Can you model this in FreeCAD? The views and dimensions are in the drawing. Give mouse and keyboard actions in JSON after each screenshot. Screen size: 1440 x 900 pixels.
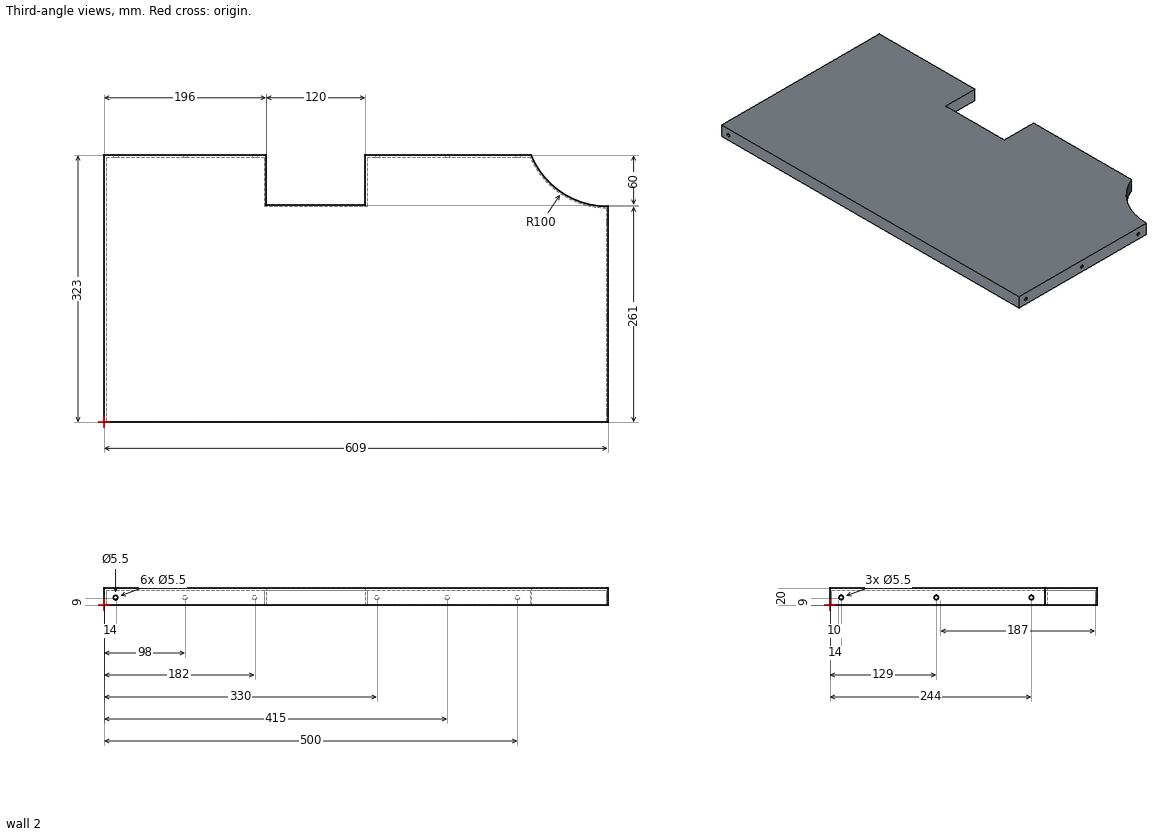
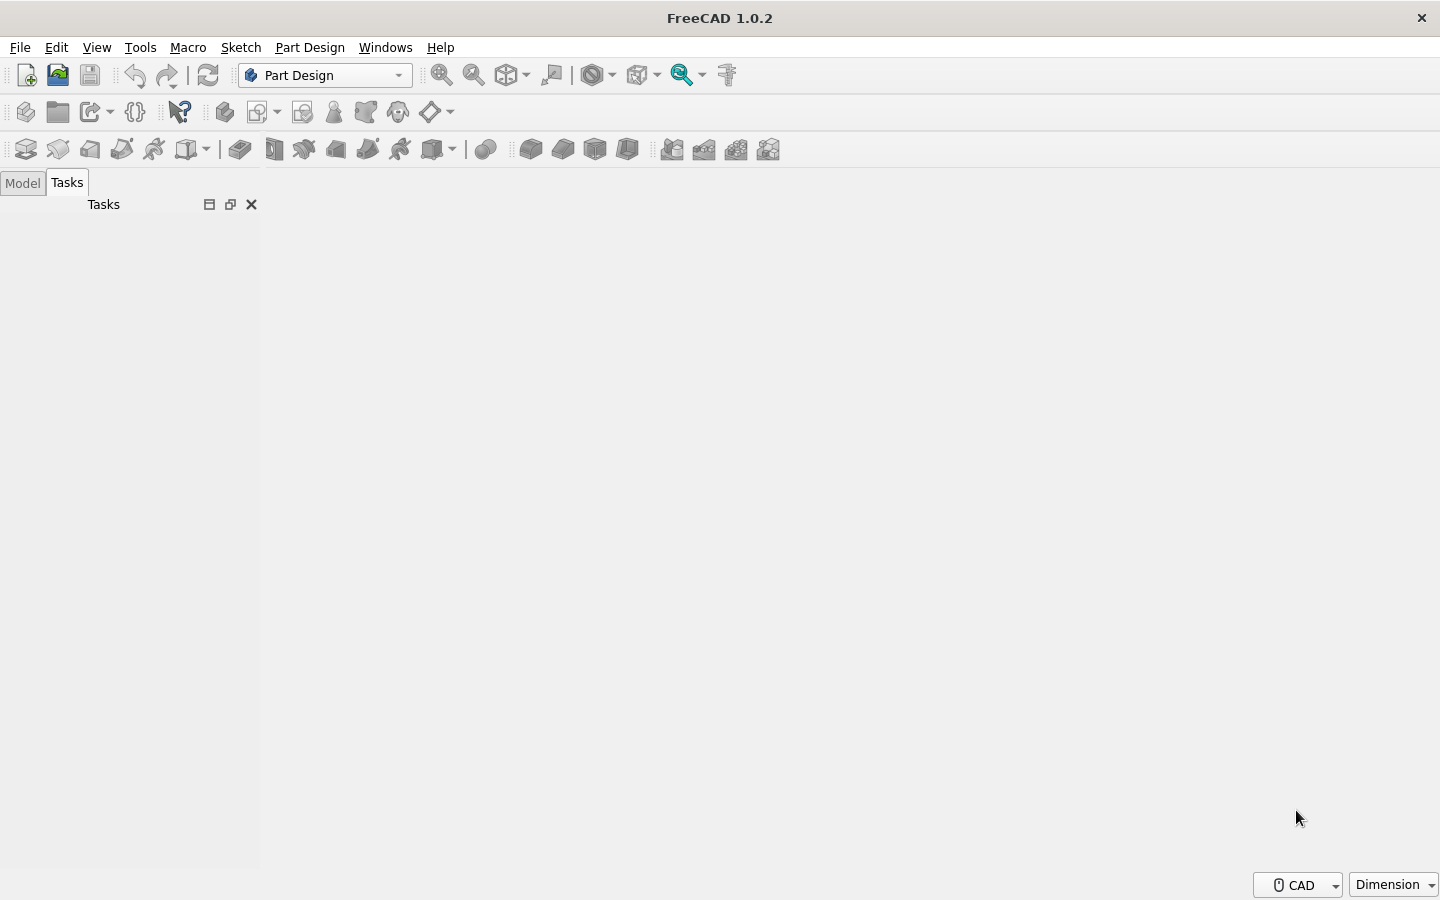
{"action": "key", "text": "ctrl+n"}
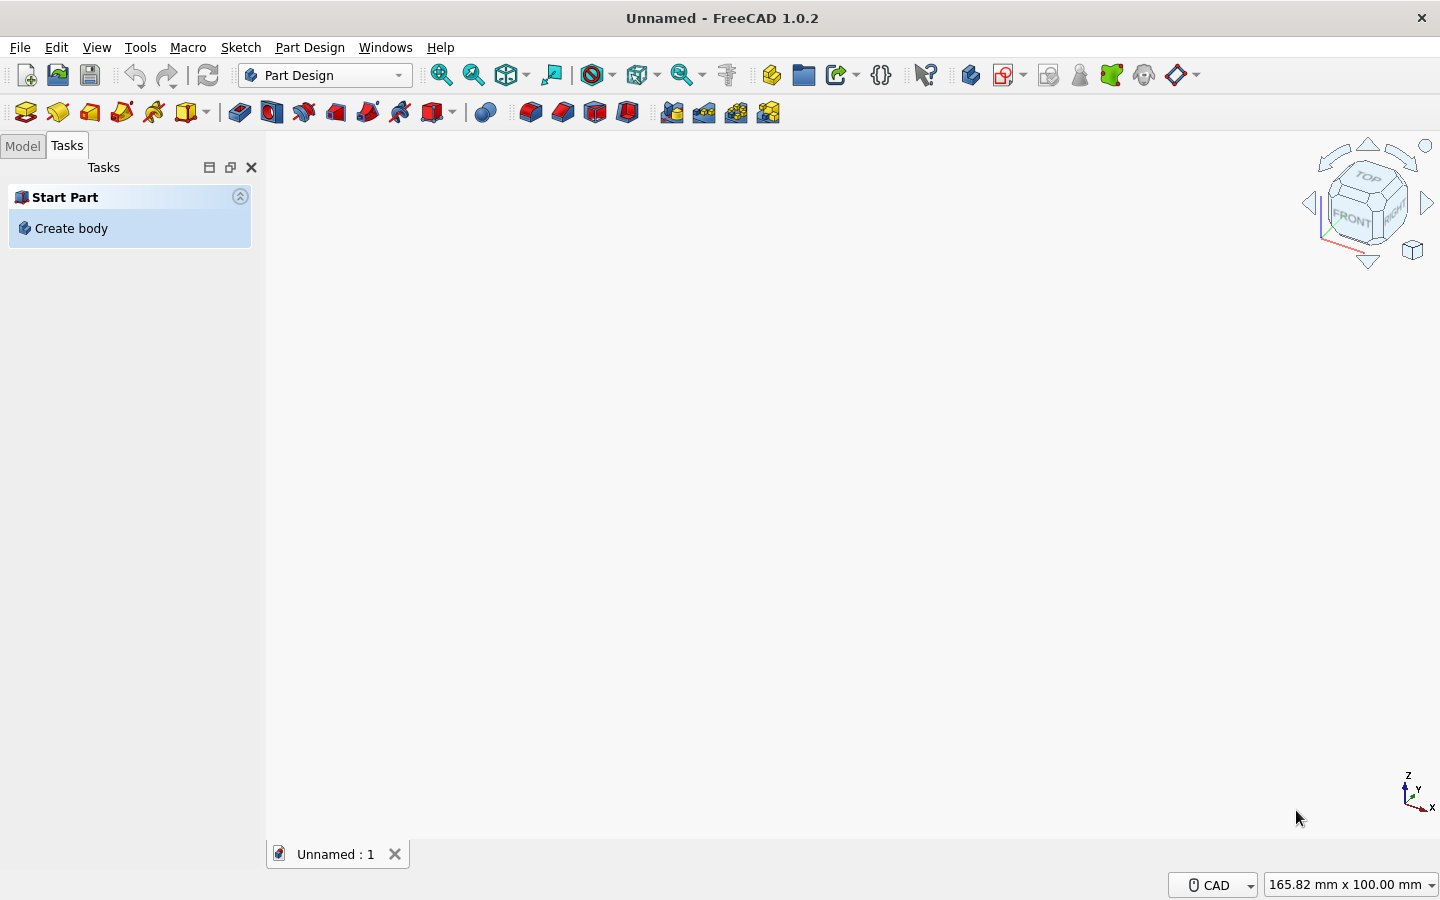
{"action": "left_click", "coordinate": [1004, 76]}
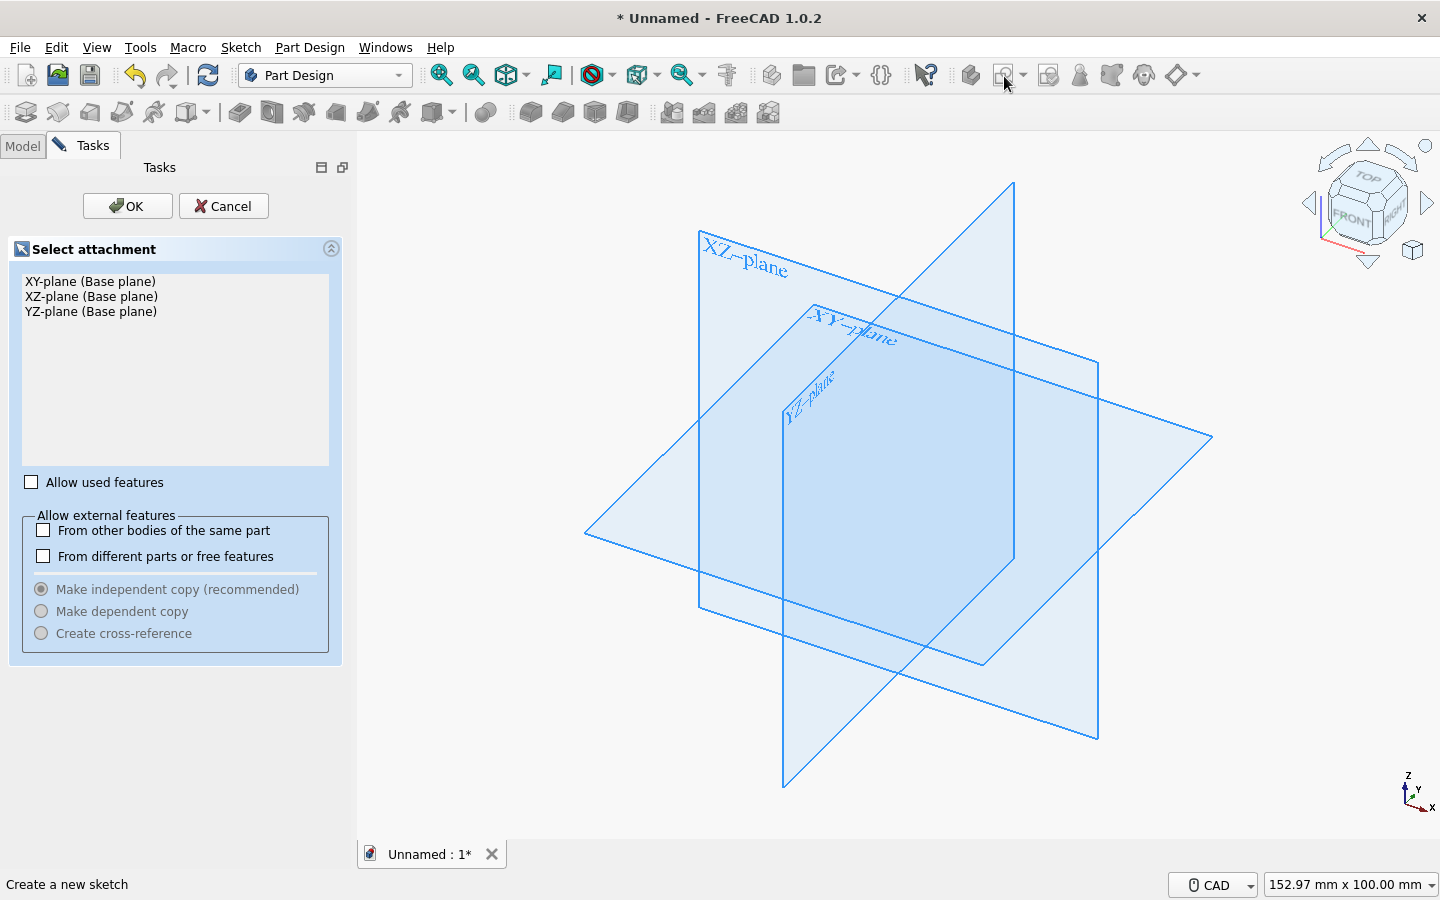
{"action": "left_click", "coordinate": [82, 282]}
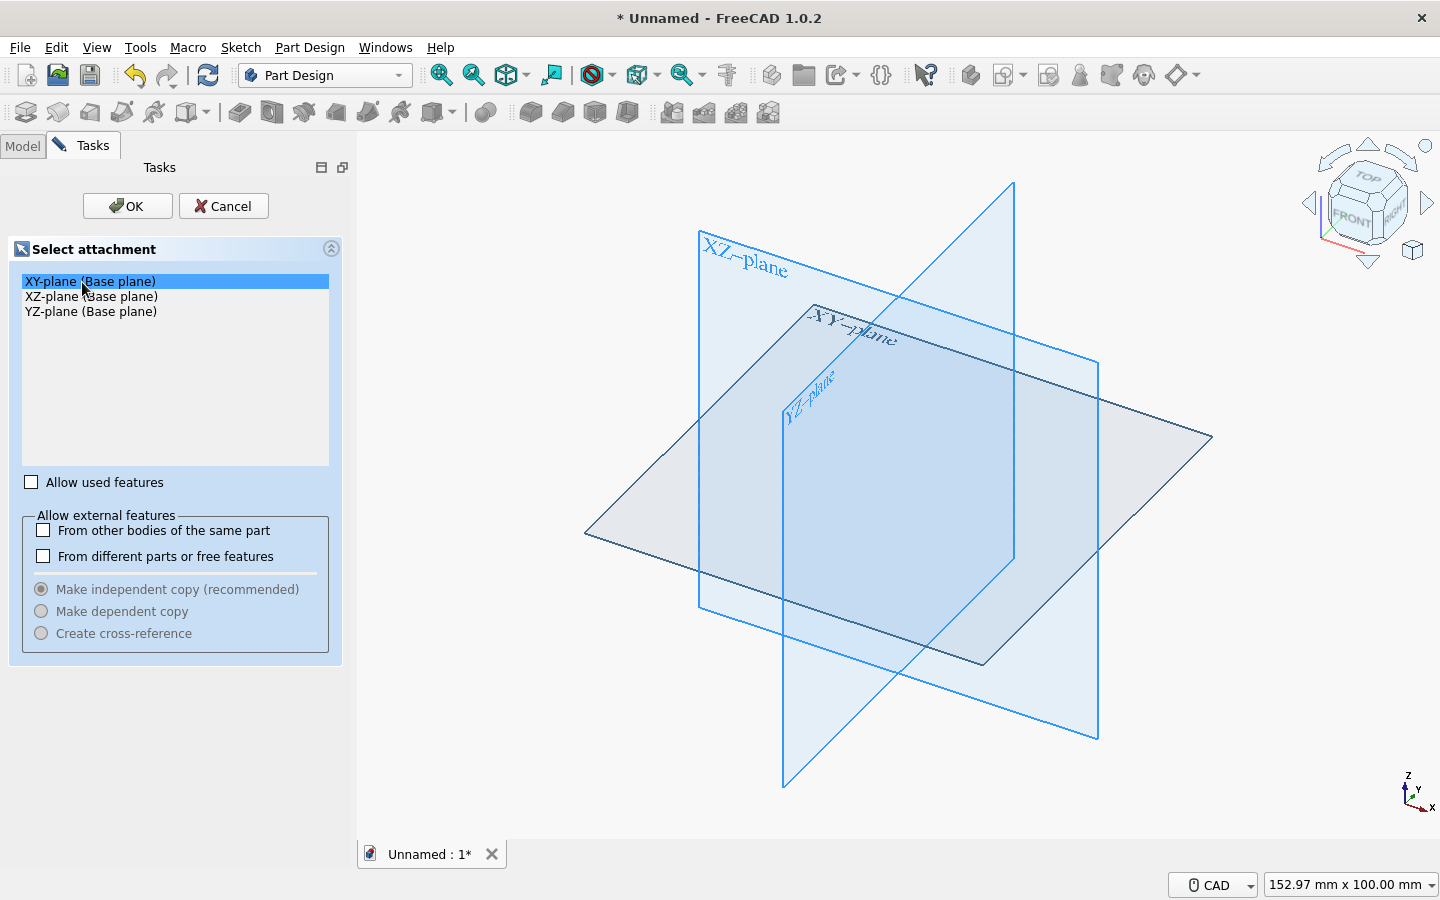
{"action": "left_click", "coordinate": [128, 206]}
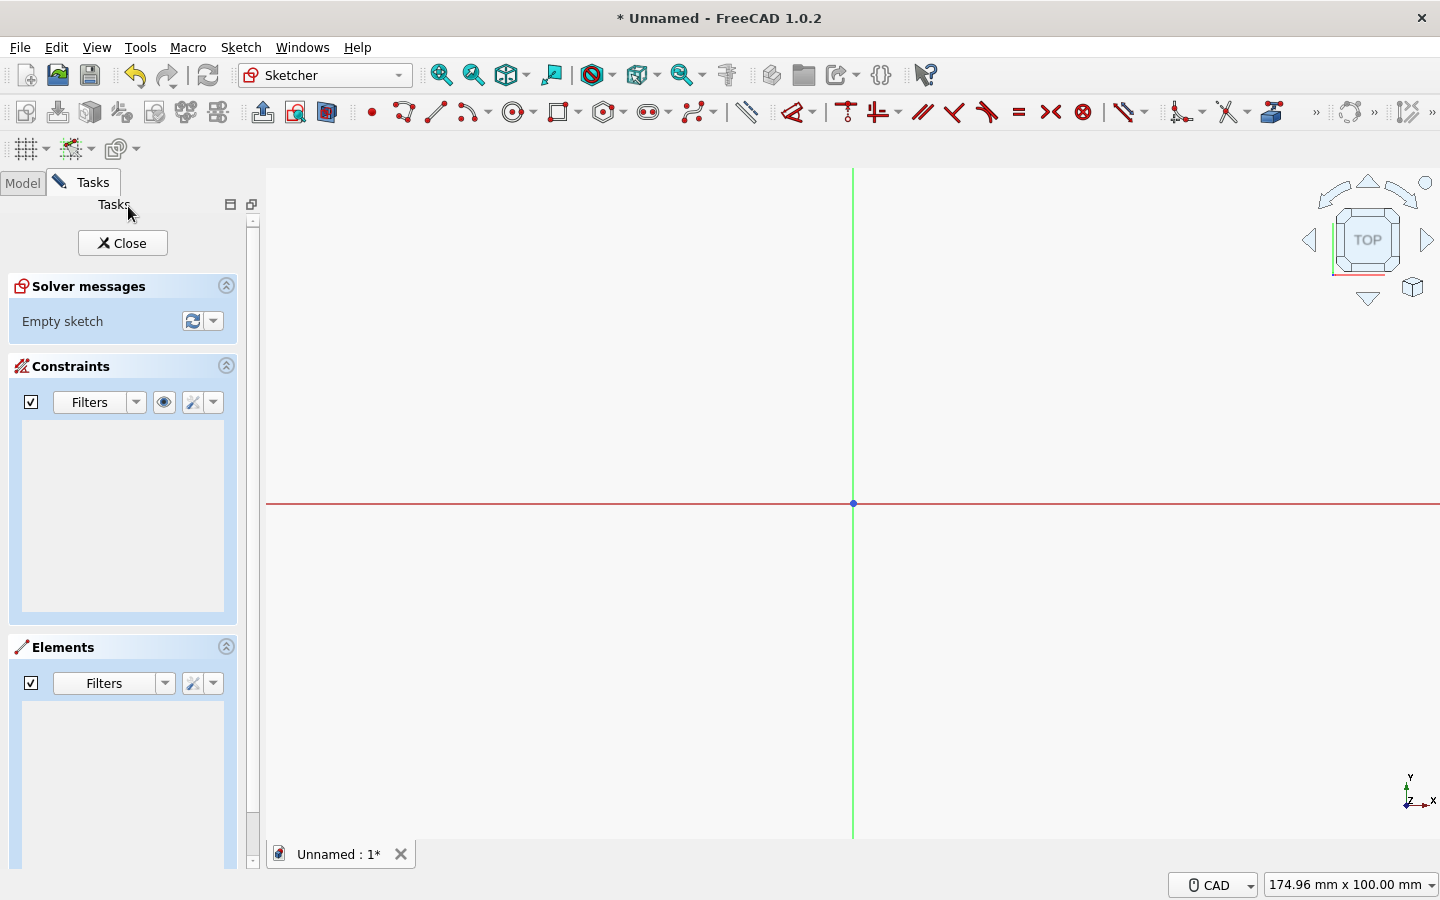
{"action": "scroll", "coordinate": [366, 718], "scroll_direction": "down", "scroll_amount": 9}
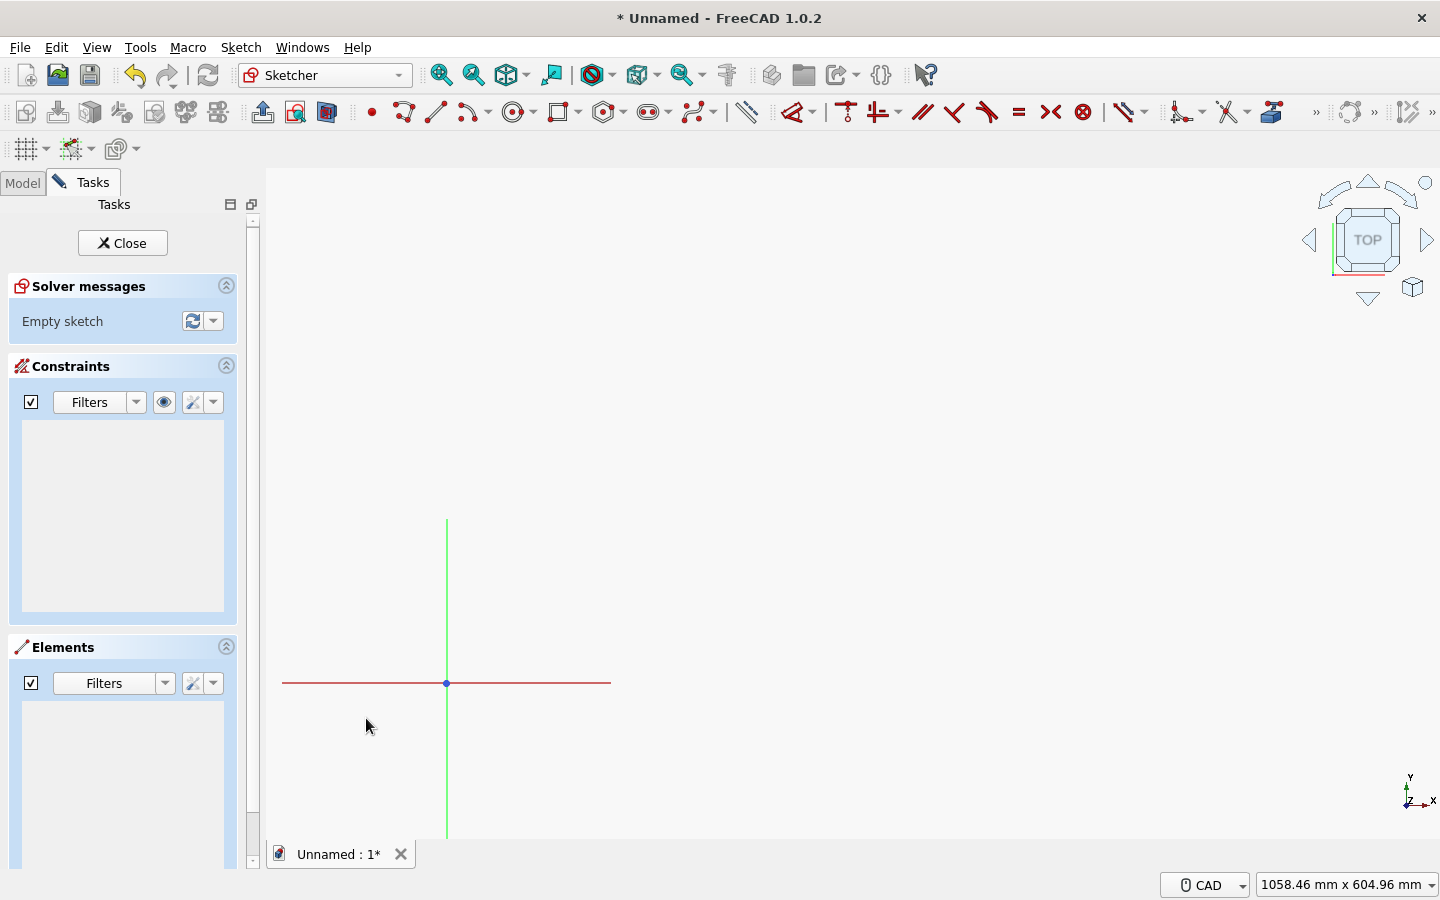
{"action": "key", "text": "g m"}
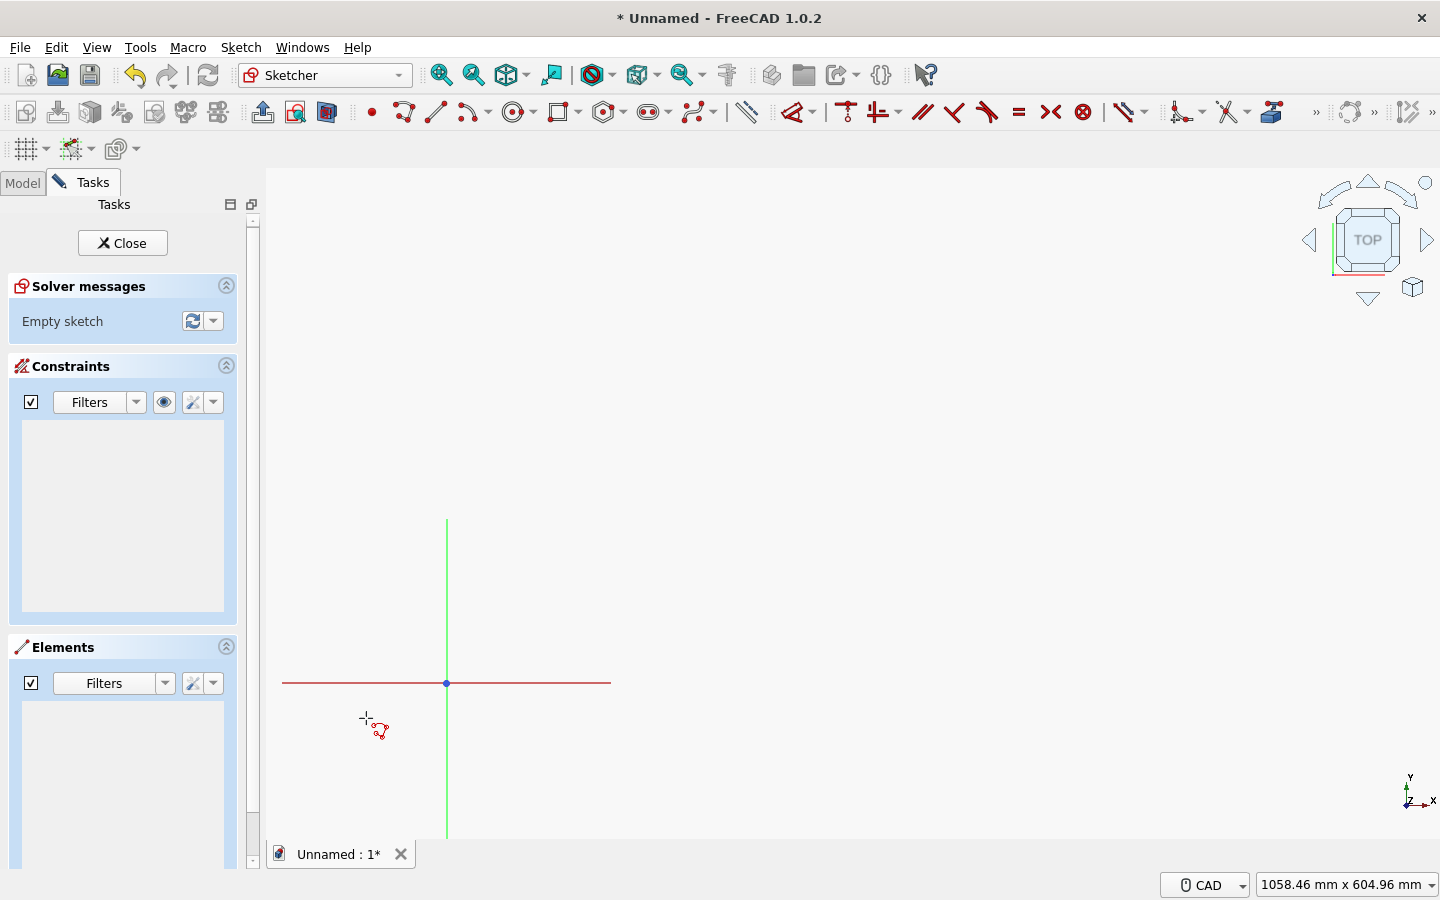
{"action": "left_click", "coordinate": [1019, 325]}
{"action": "left_click", "coordinate": [797, 325]}
{"action": "left_click", "coordinate": [797, 392]}
{"action": "left_click", "coordinate": [664, 392]}
{"action": "left_click", "coordinate": [664, 325]}
{"action": "left_click", "coordinate": [447, 325]}
{"action": "left_click", "coordinate": [447, 683]}
{"action": "left_click", "coordinate": [1122, 674]}
{"action": "left_click", "coordinate": [1122, 394]}
{"action": "right_click", "coordinate": [1122, 394]}